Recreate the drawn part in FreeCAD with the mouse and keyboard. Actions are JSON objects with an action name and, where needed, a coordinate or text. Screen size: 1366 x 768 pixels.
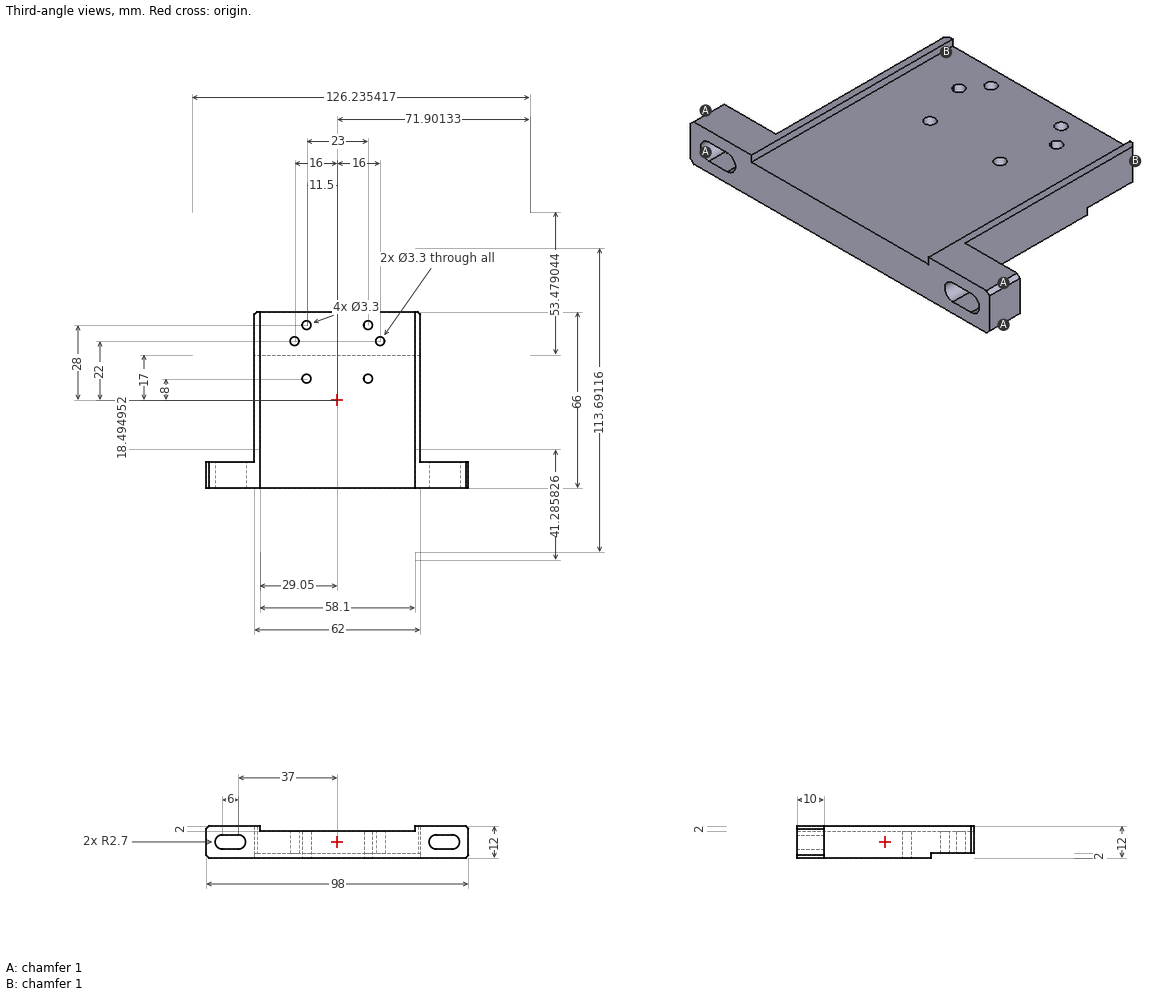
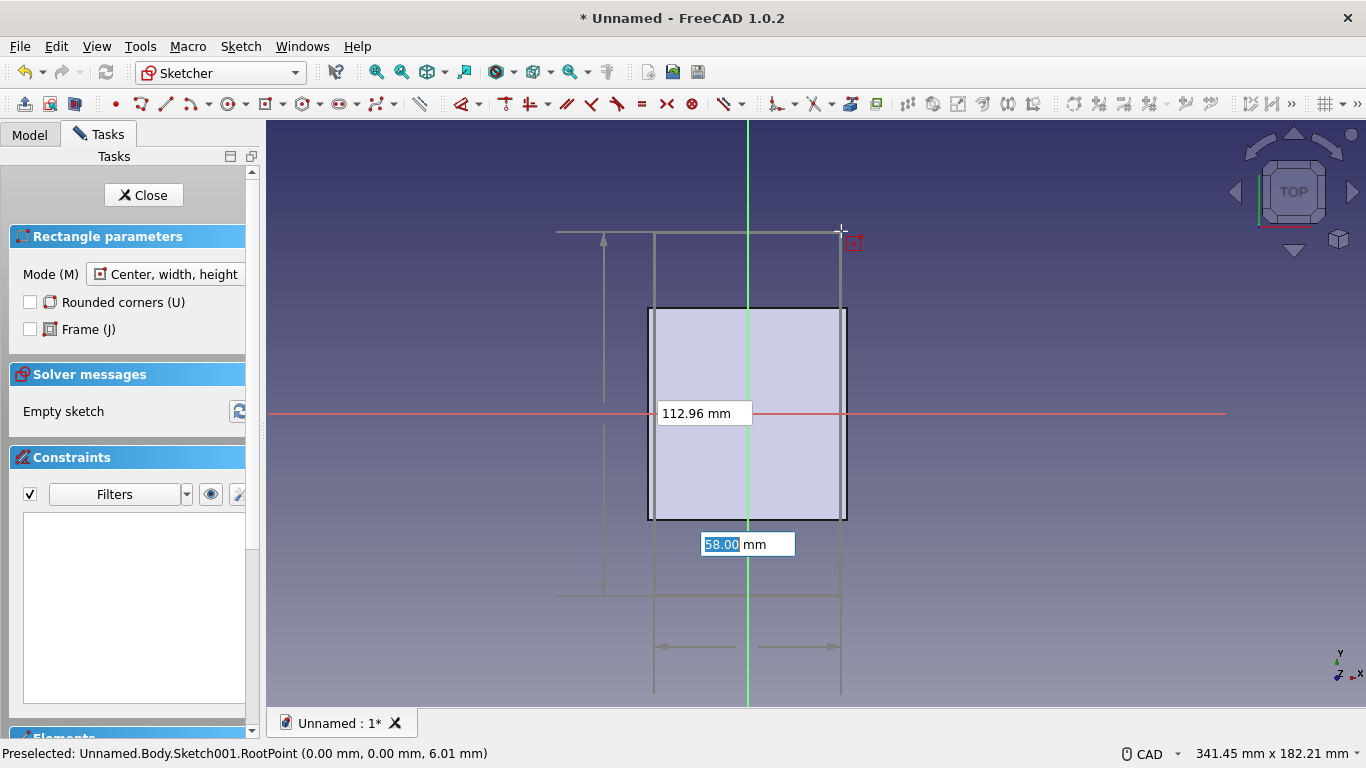
{"action": "type", "text": "58.1"}
{"action": "key", "text": "Tab"}
{"action": "type", "text": "113.69116"}
{"action": "key", "text": "Return"}
{"action": "key", "text": "Escape"}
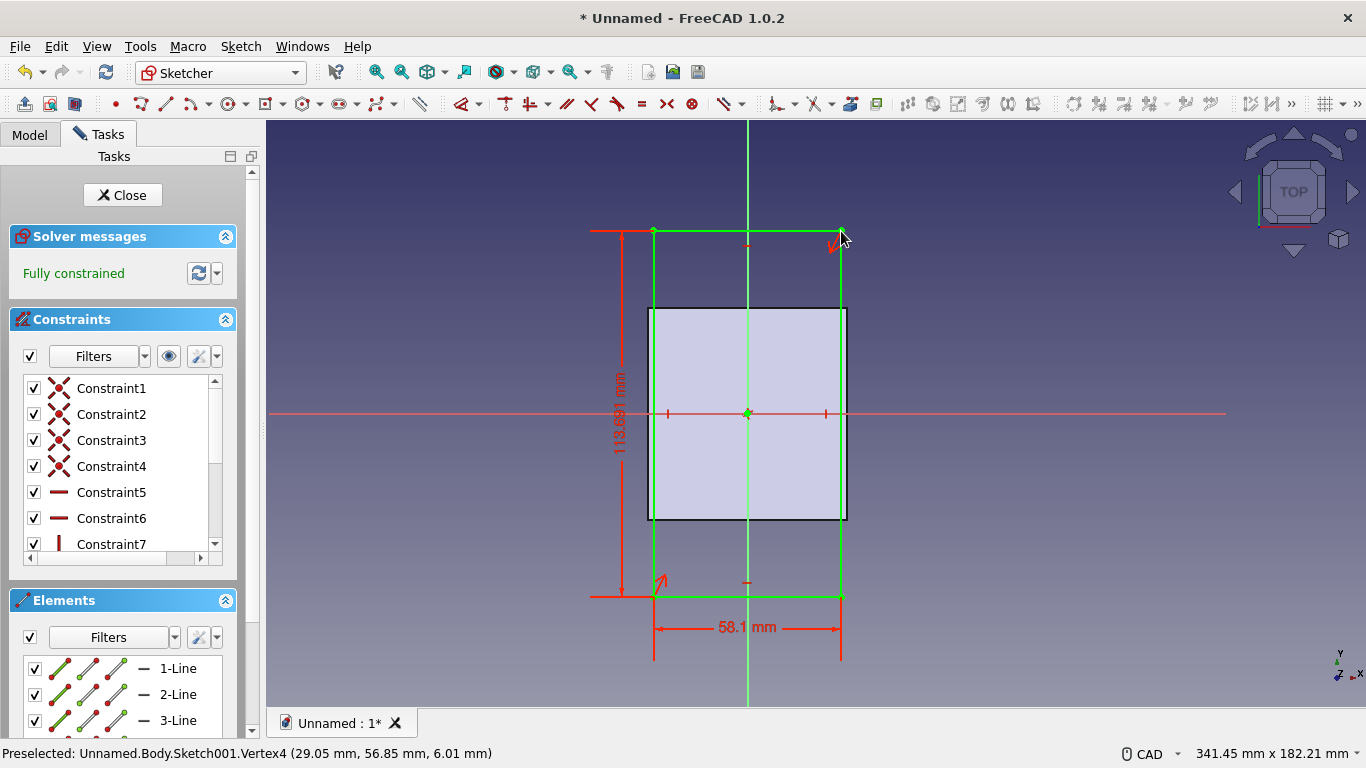
{"action": "left_click", "coordinate": [123, 195]}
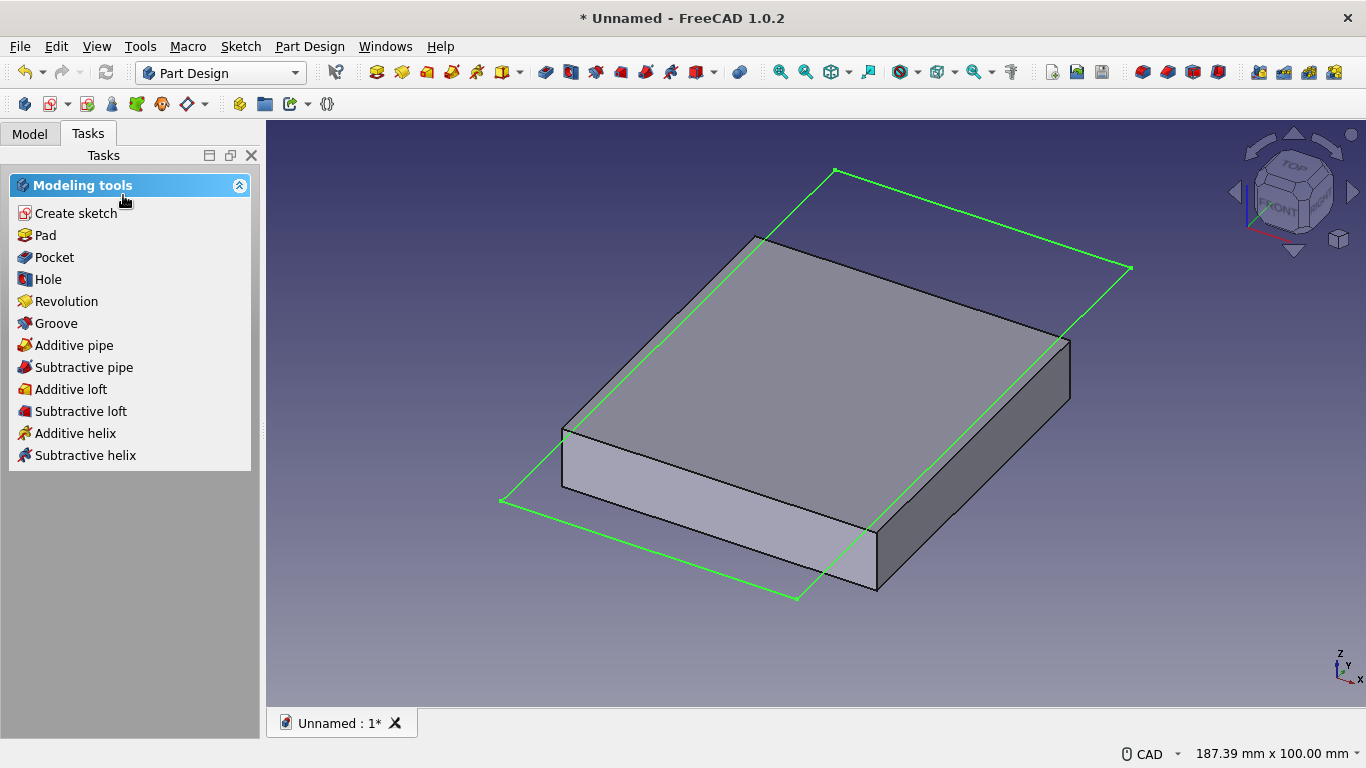
{"action": "left_click", "coordinate": [546, 72]}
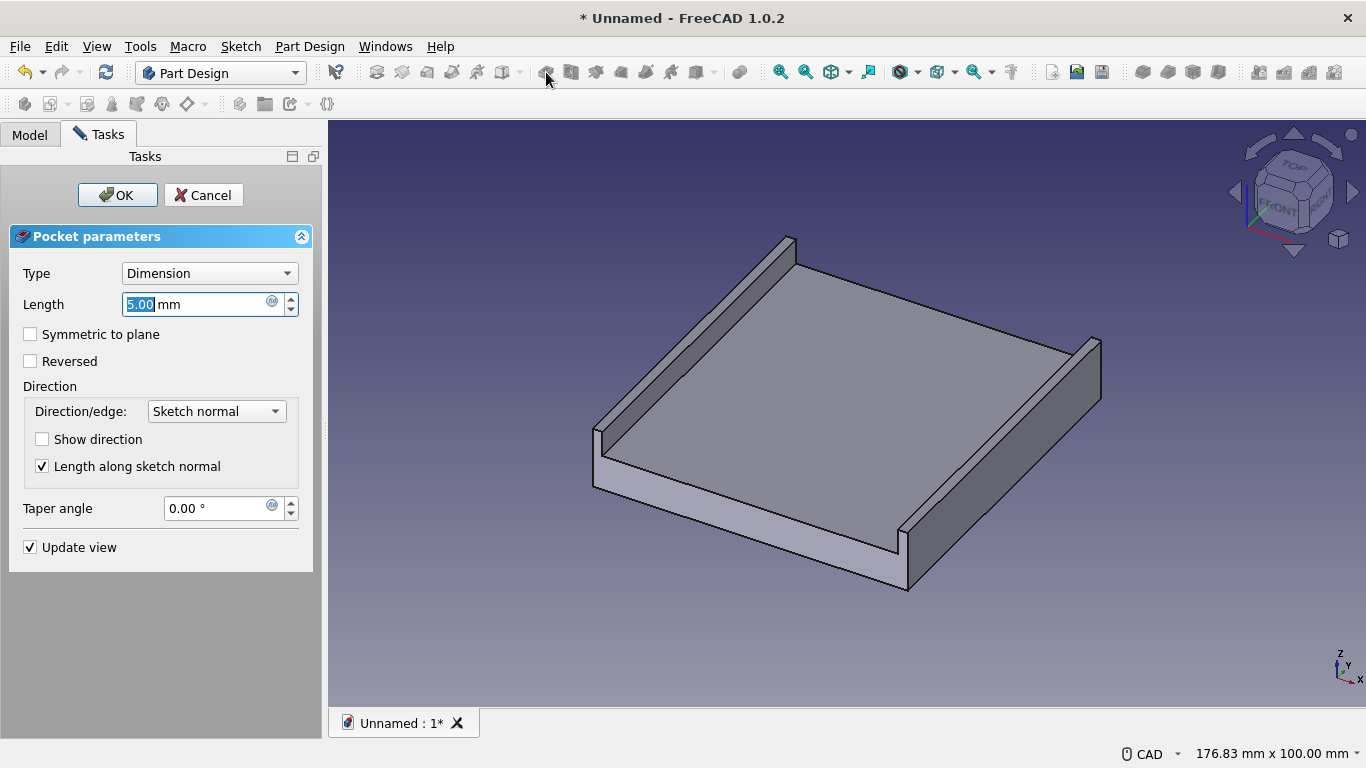
{"action": "type", "text": "2"}
{"action": "key", "text": "Tab"}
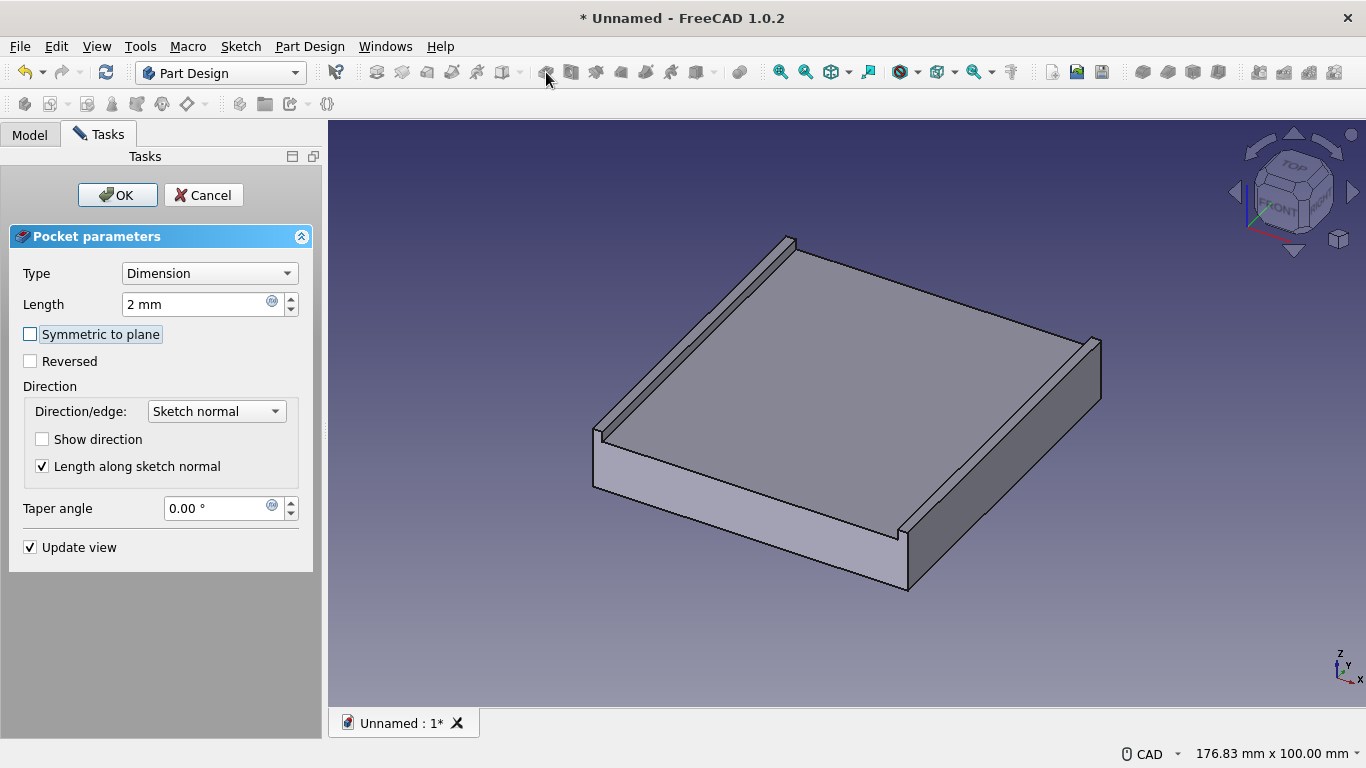
{"action": "left_click", "coordinate": [118, 195]}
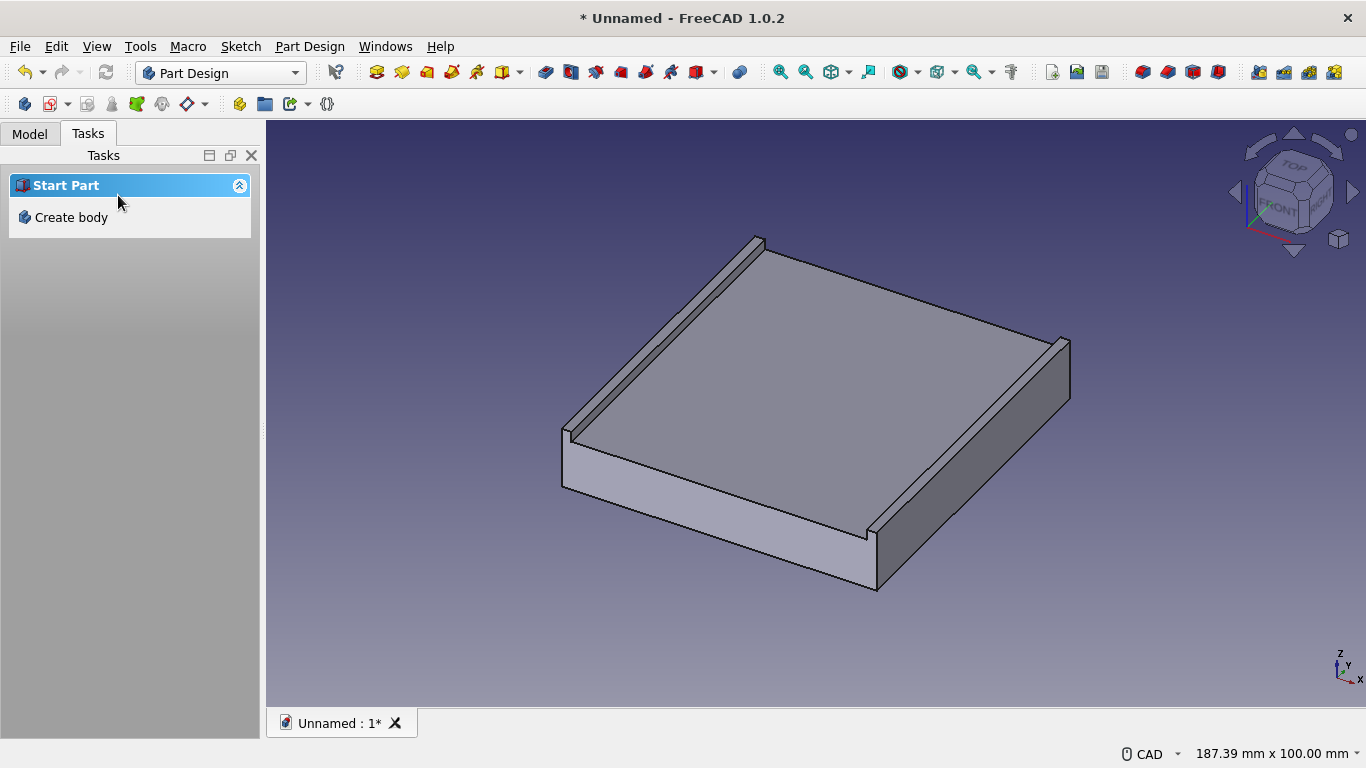
{"action": "left_click", "coordinate": [816, 393]}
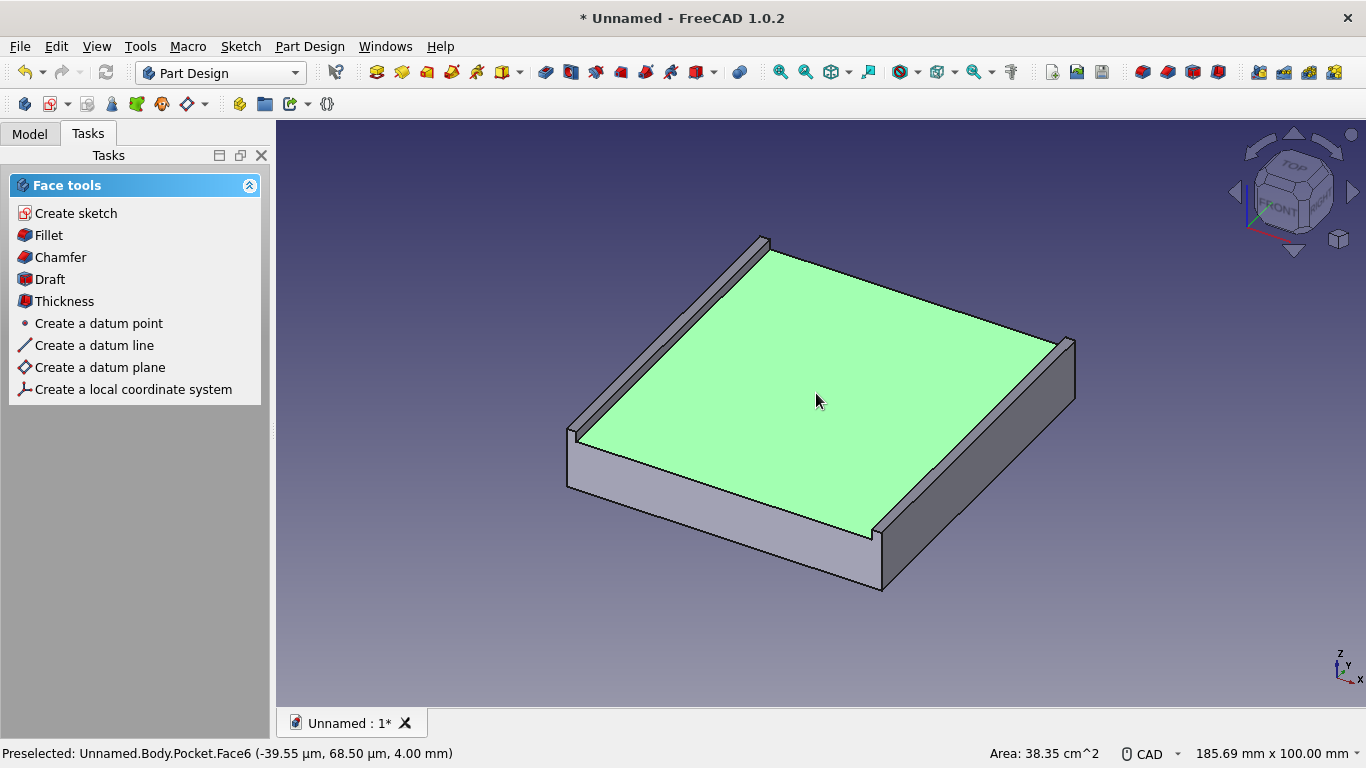
{"action": "left_click", "coordinate": [50, 104]}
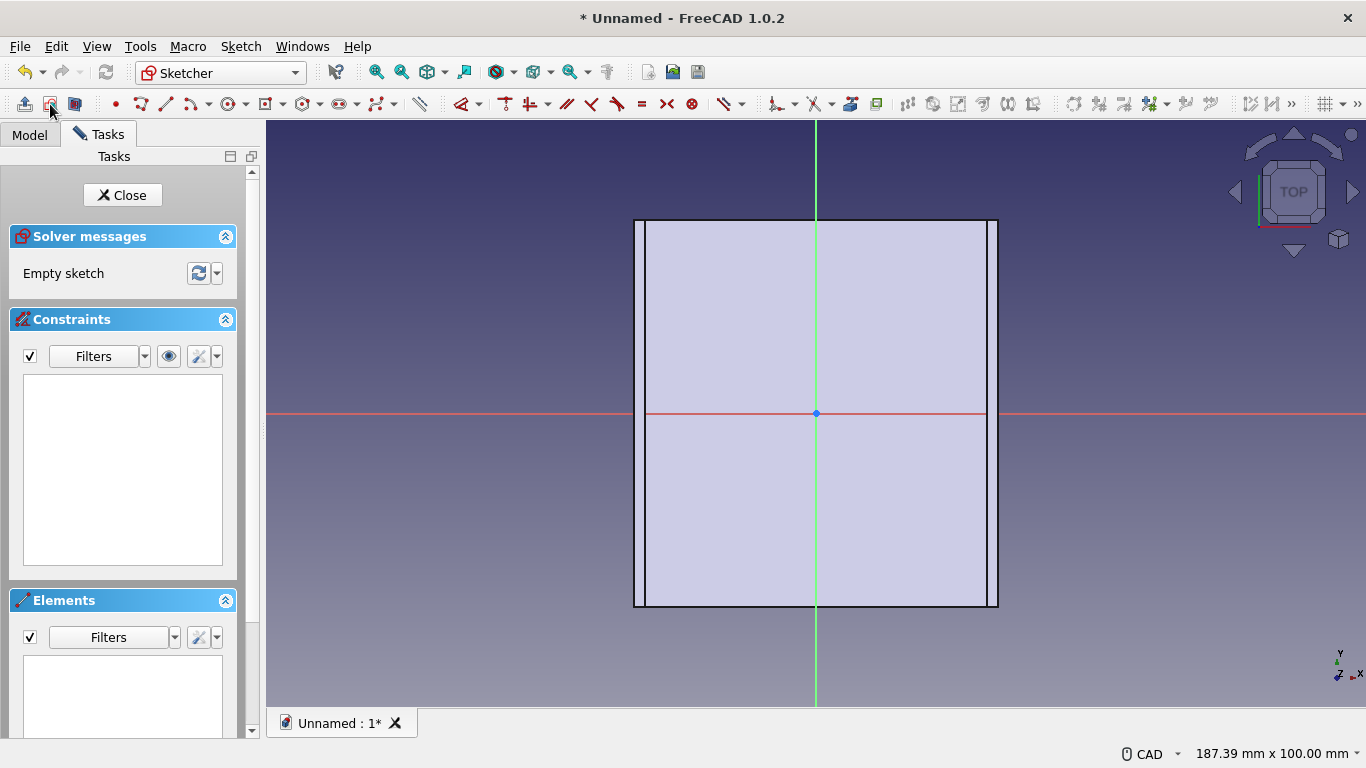
{"action": "left_click", "coordinate": [75, 104]}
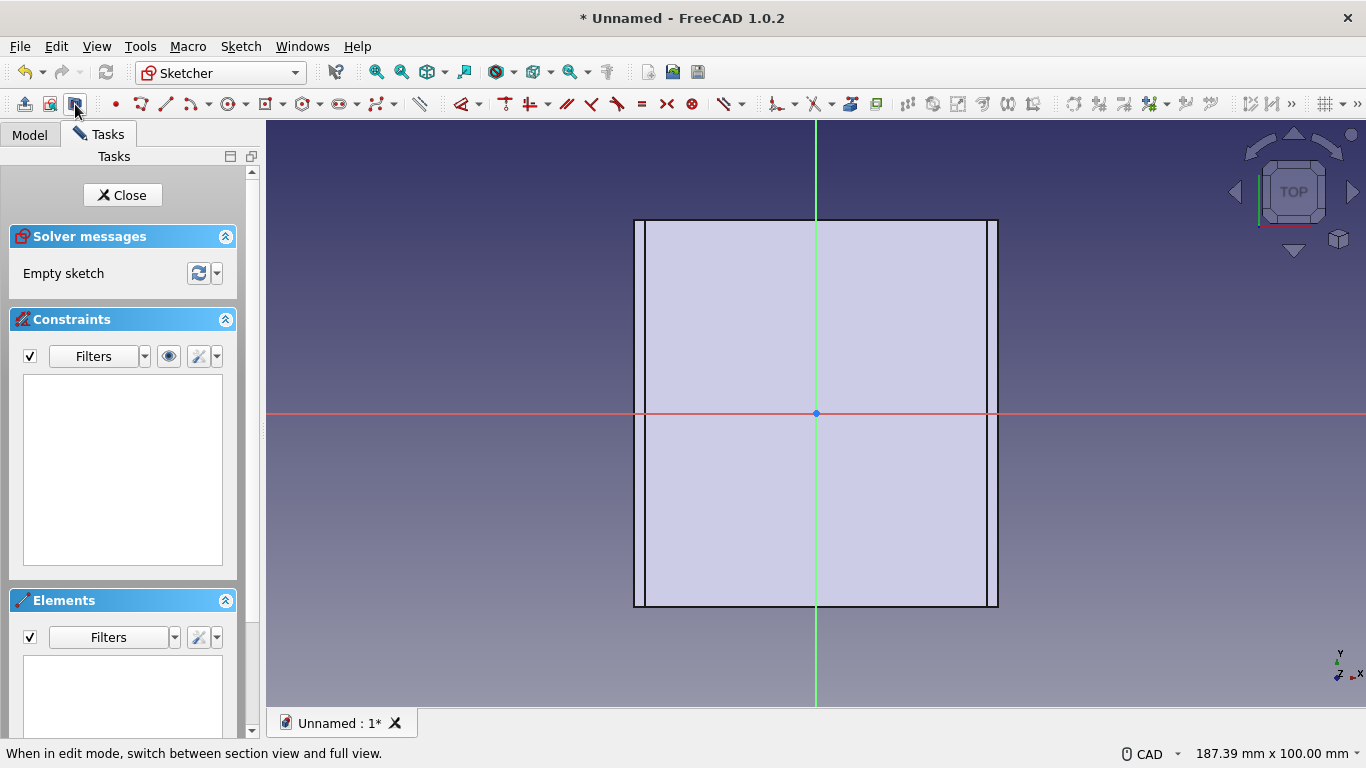
{"action": "scroll", "coordinate": [872, 255], "scroll_direction": "up", "scroll_amount": 4}